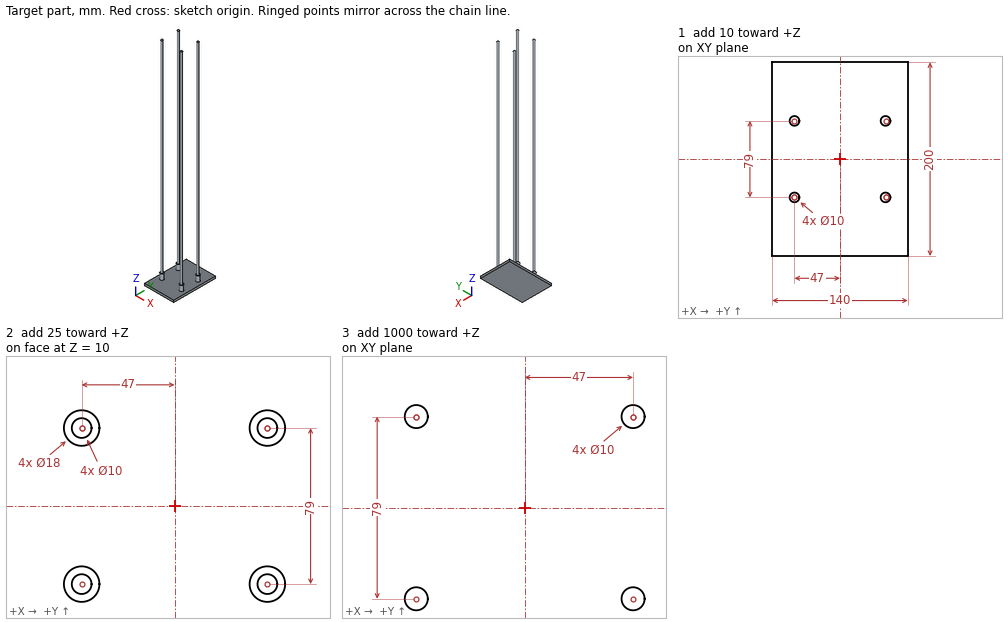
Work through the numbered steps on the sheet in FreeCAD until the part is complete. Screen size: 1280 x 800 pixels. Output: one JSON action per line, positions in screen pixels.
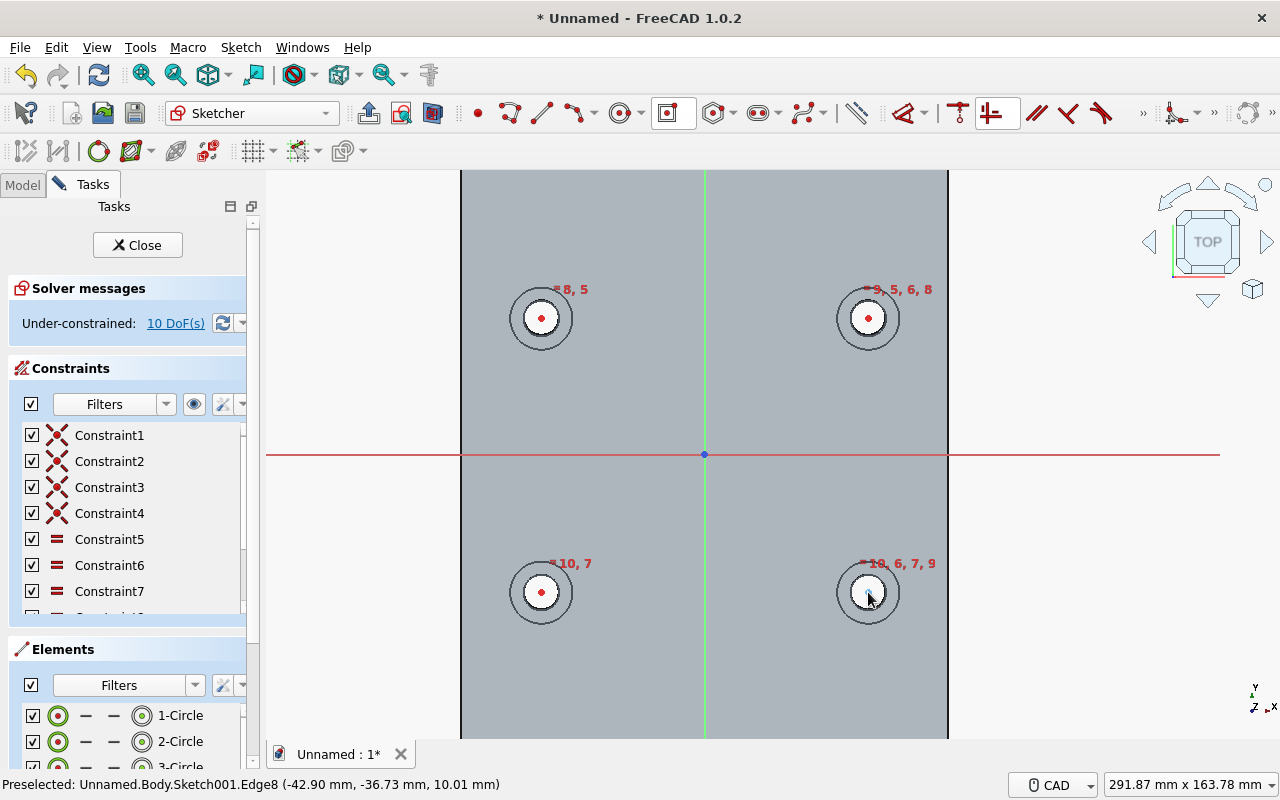
{"action": "left_click", "coordinate": [541, 319]}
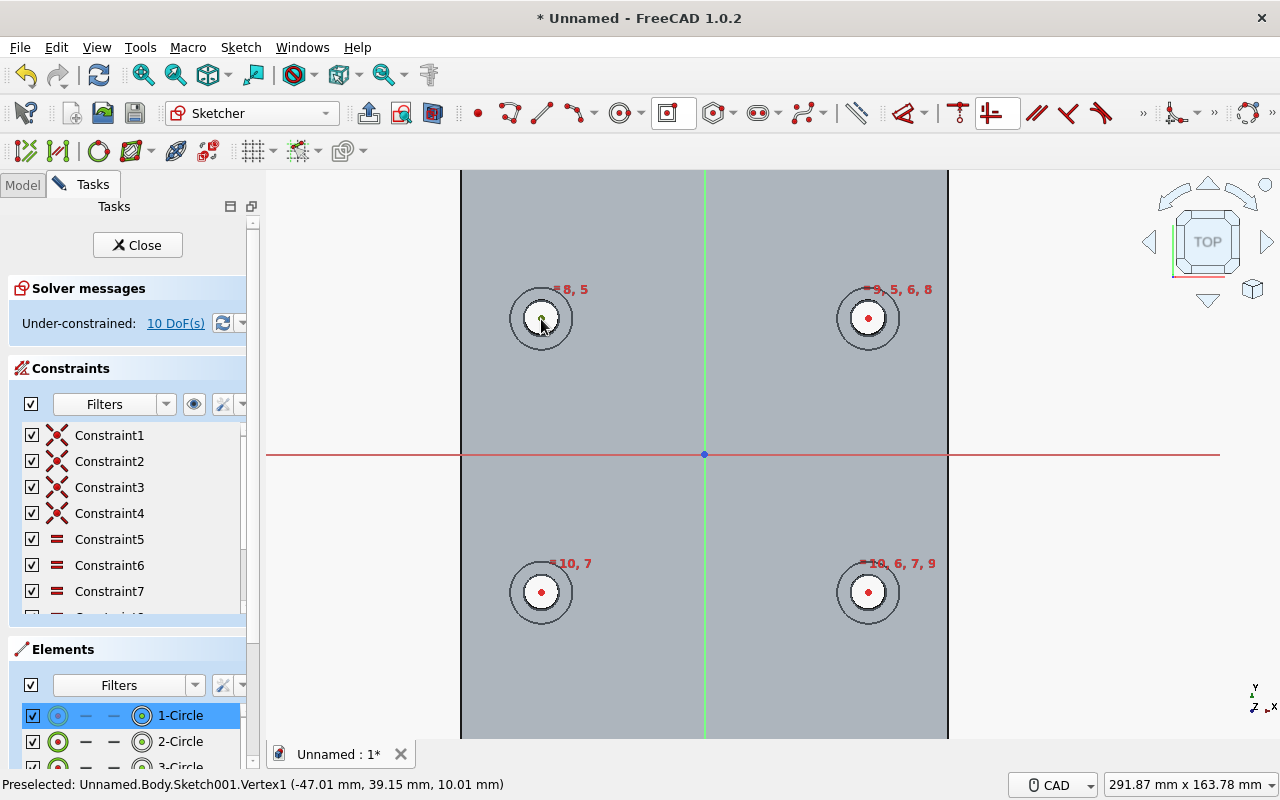
{"action": "left_click", "coordinate": [868, 319]}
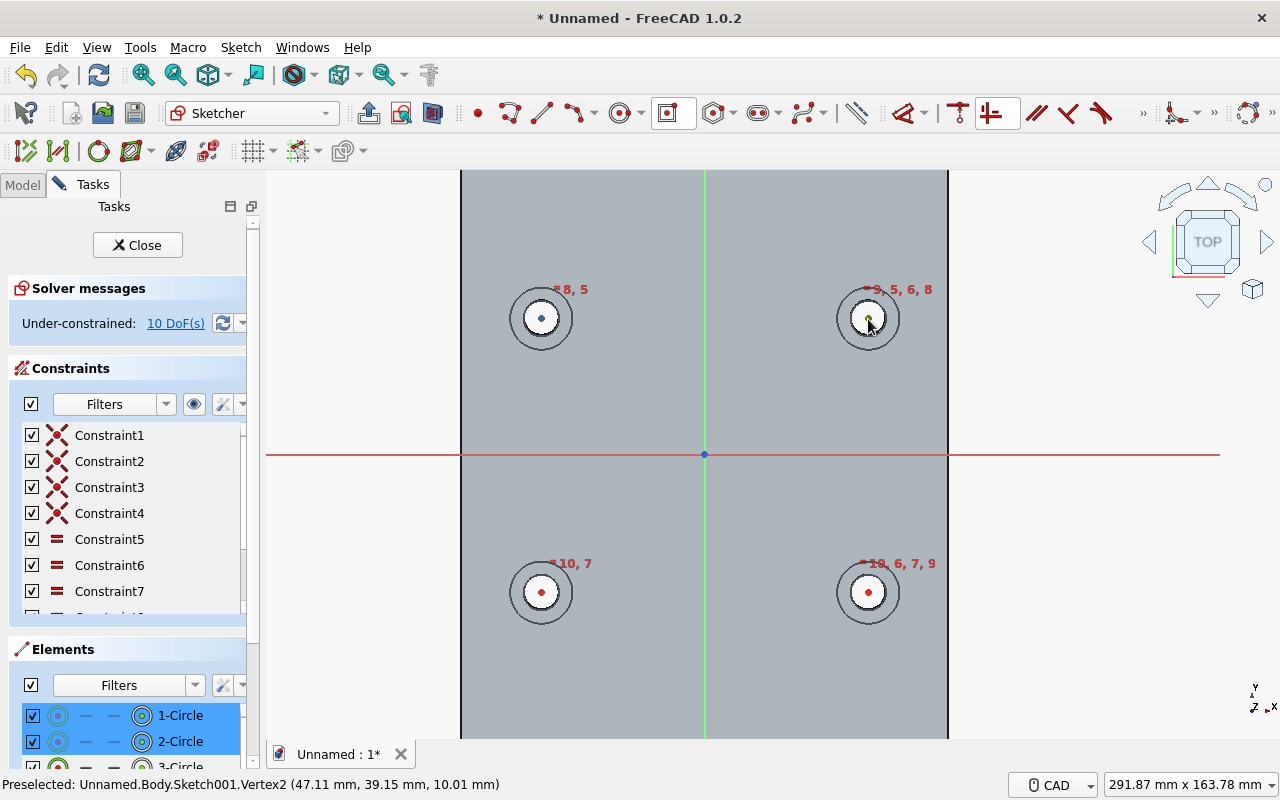
{"action": "left_click", "coordinate": [705, 674]}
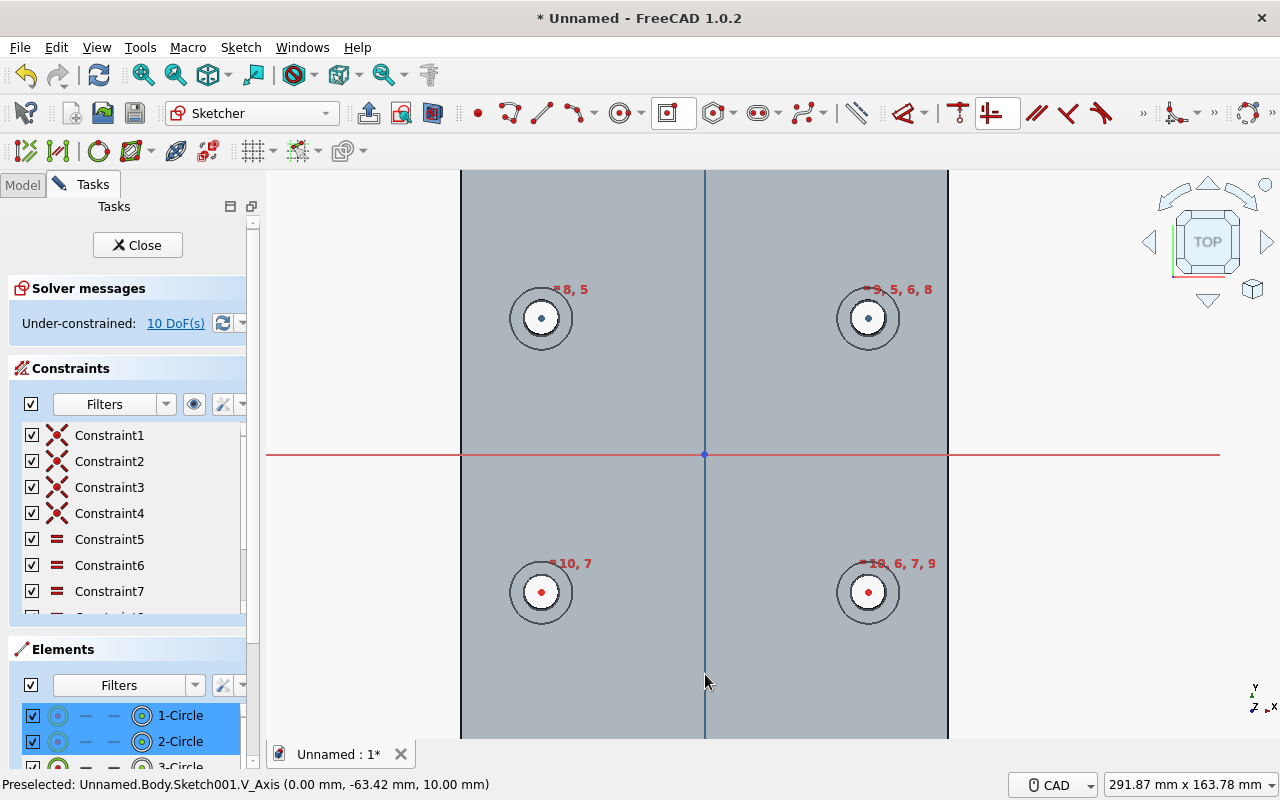
{"action": "key", "text": "s"}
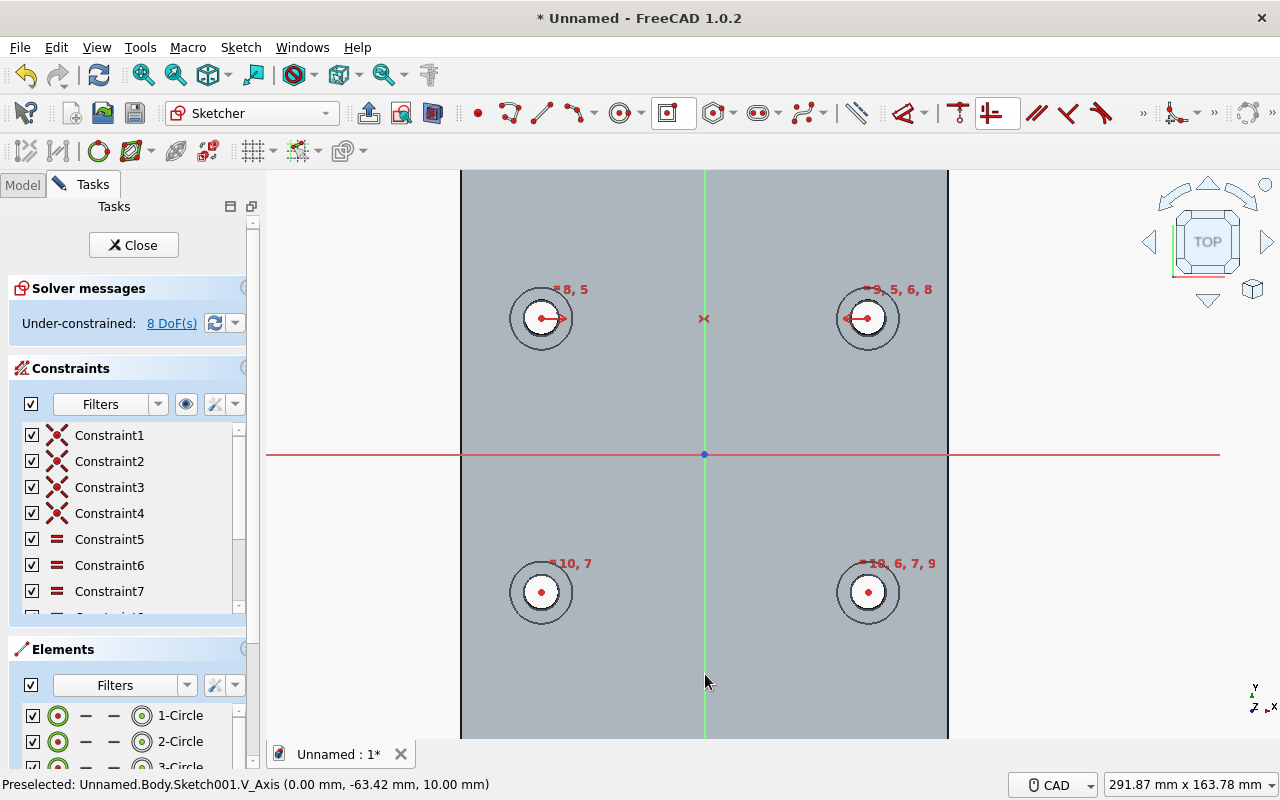
{"action": "left_click", "coordinate": [868, 319]}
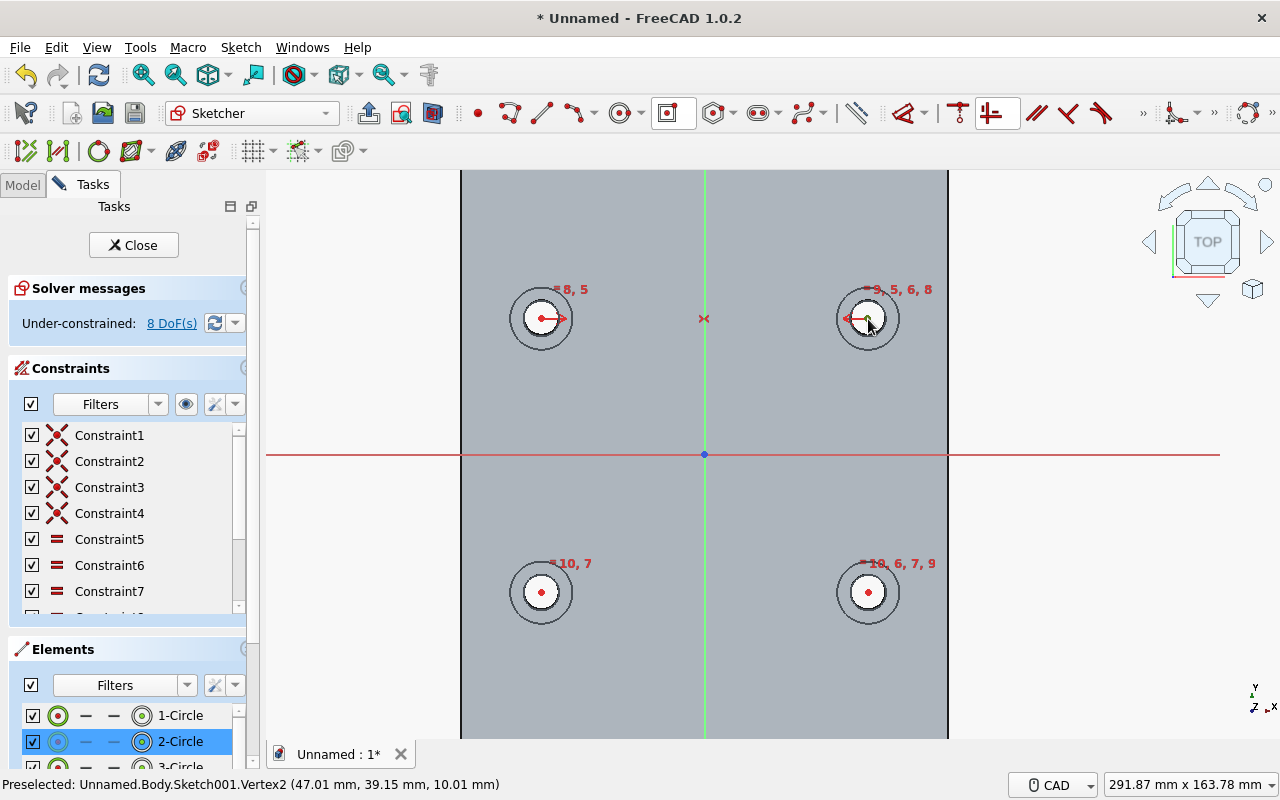
{"action": "left_click", "coordinate": [868, 593]}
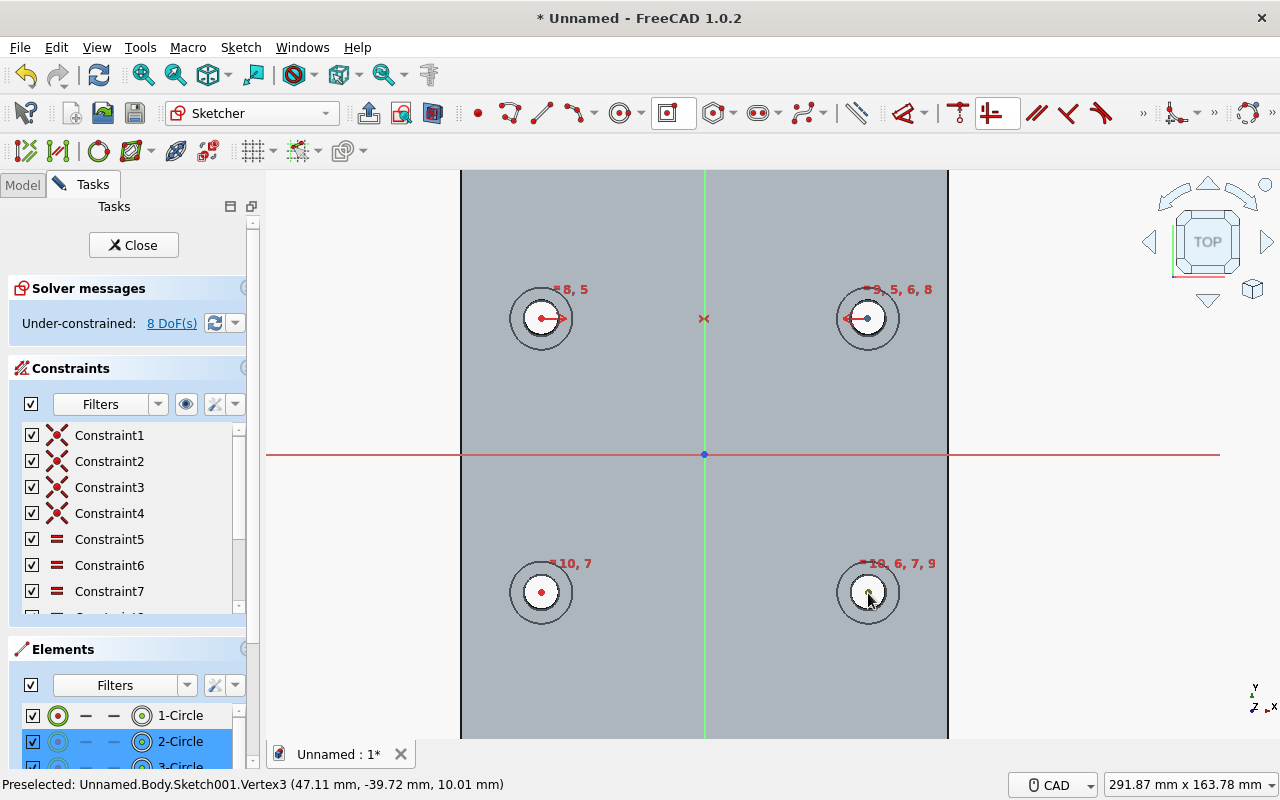
{"action": "left_click", "coordinate": [353, 455]}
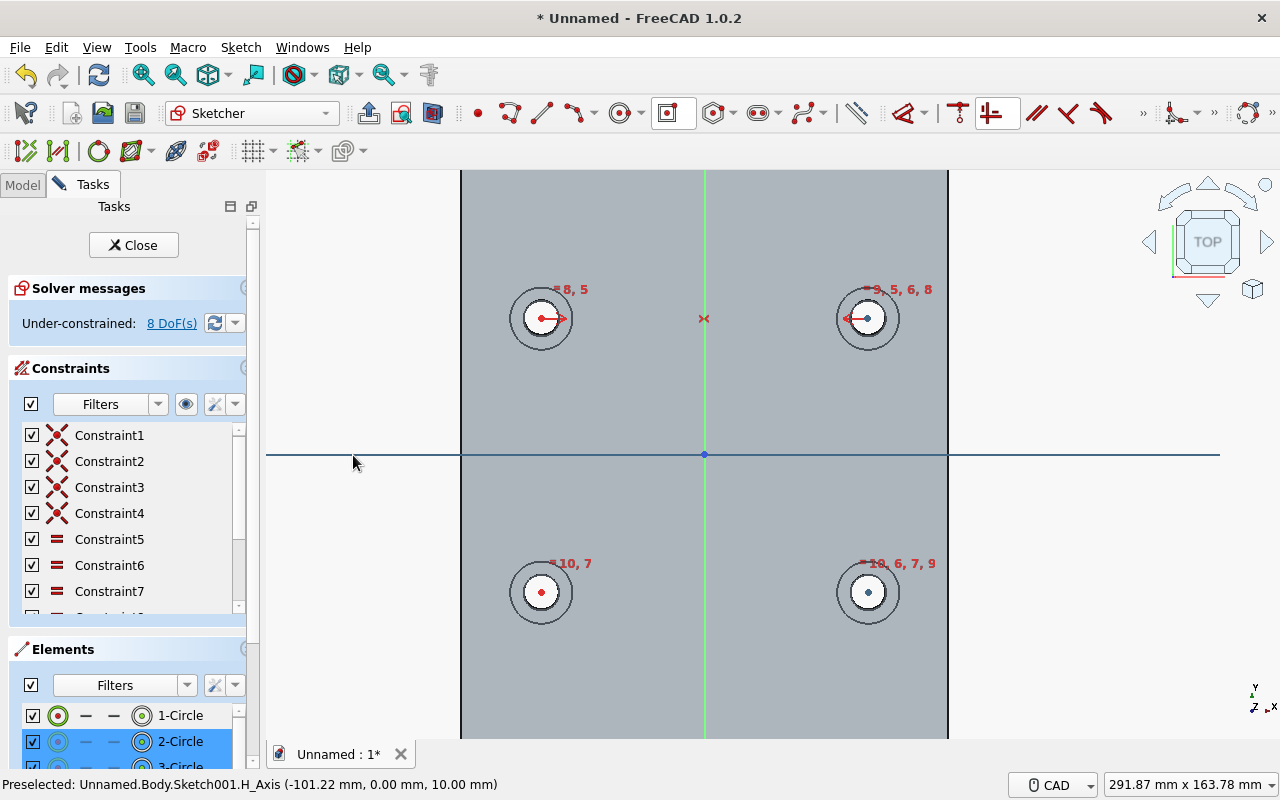
{"action": "key", "text": "s"}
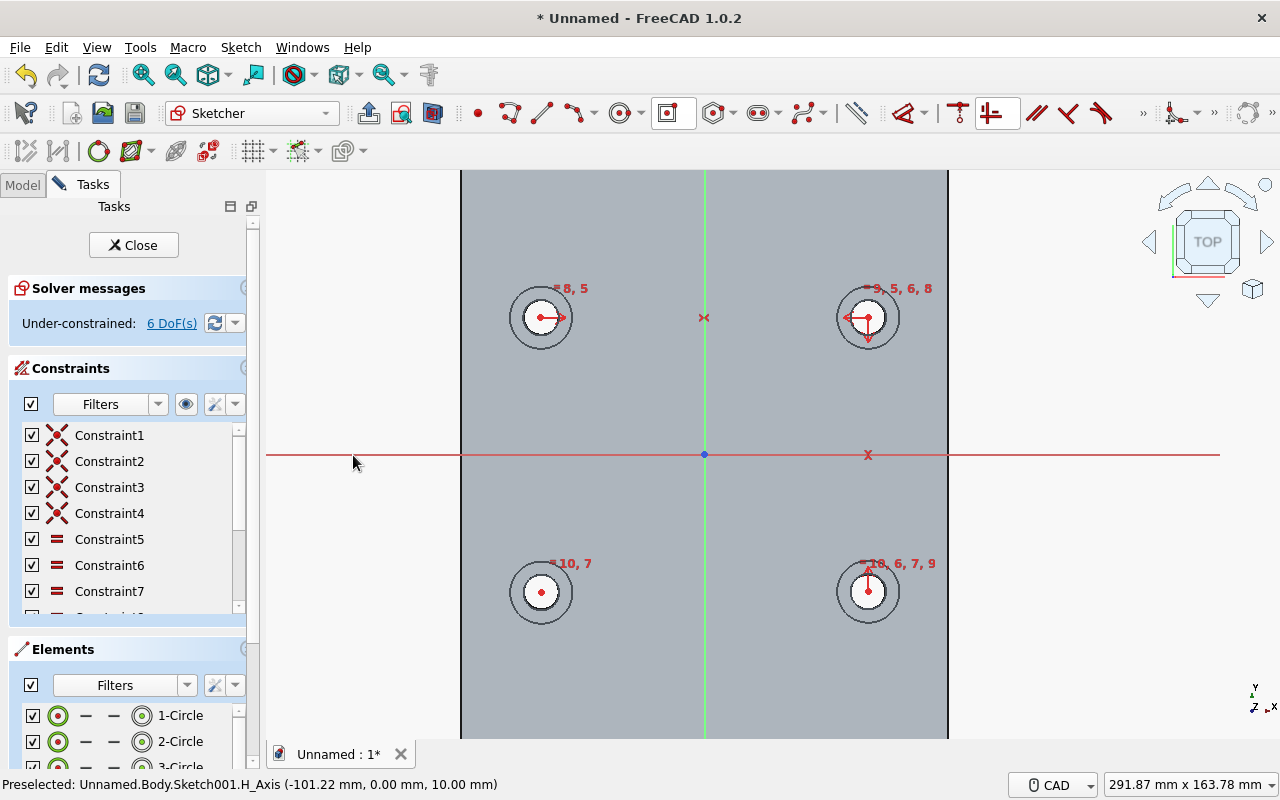
{"action": "left_click", "coordinate": [541, 318]}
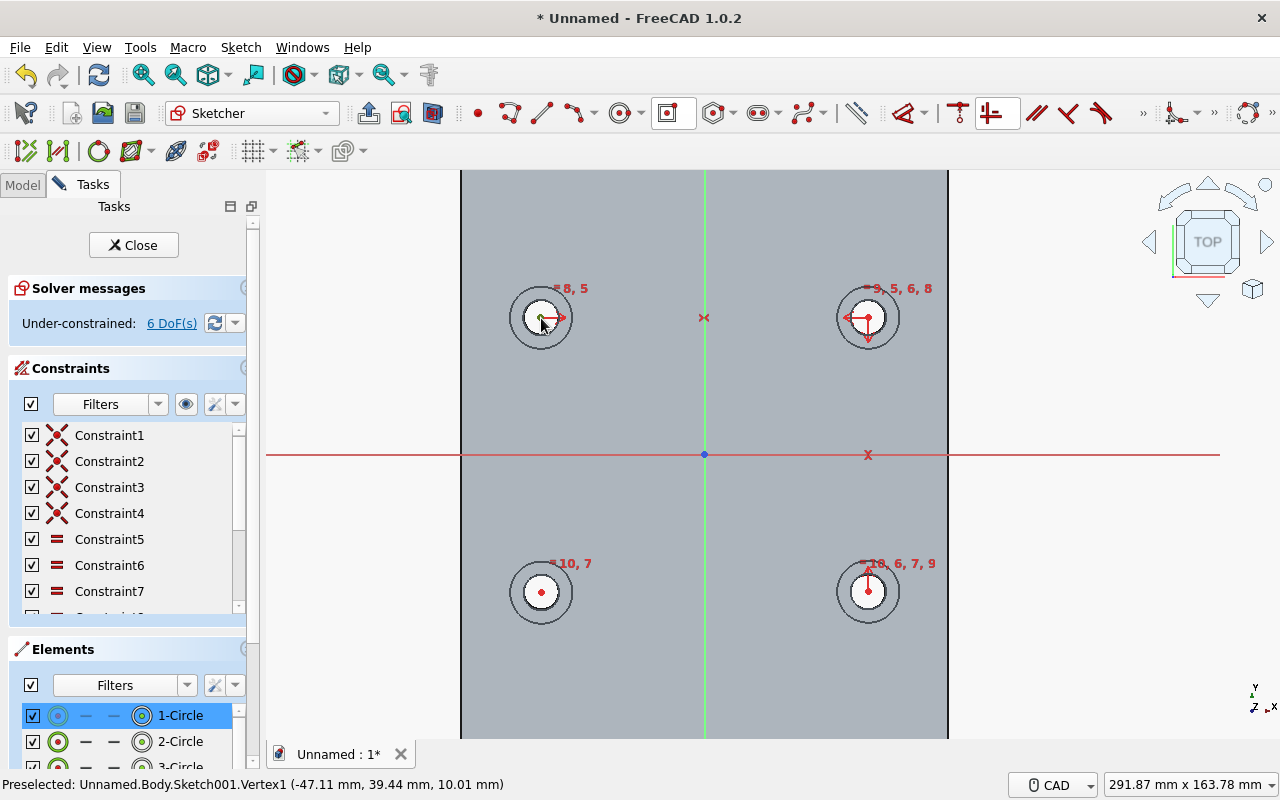
{"action": "left_click", "coordinate": [541, 593]}